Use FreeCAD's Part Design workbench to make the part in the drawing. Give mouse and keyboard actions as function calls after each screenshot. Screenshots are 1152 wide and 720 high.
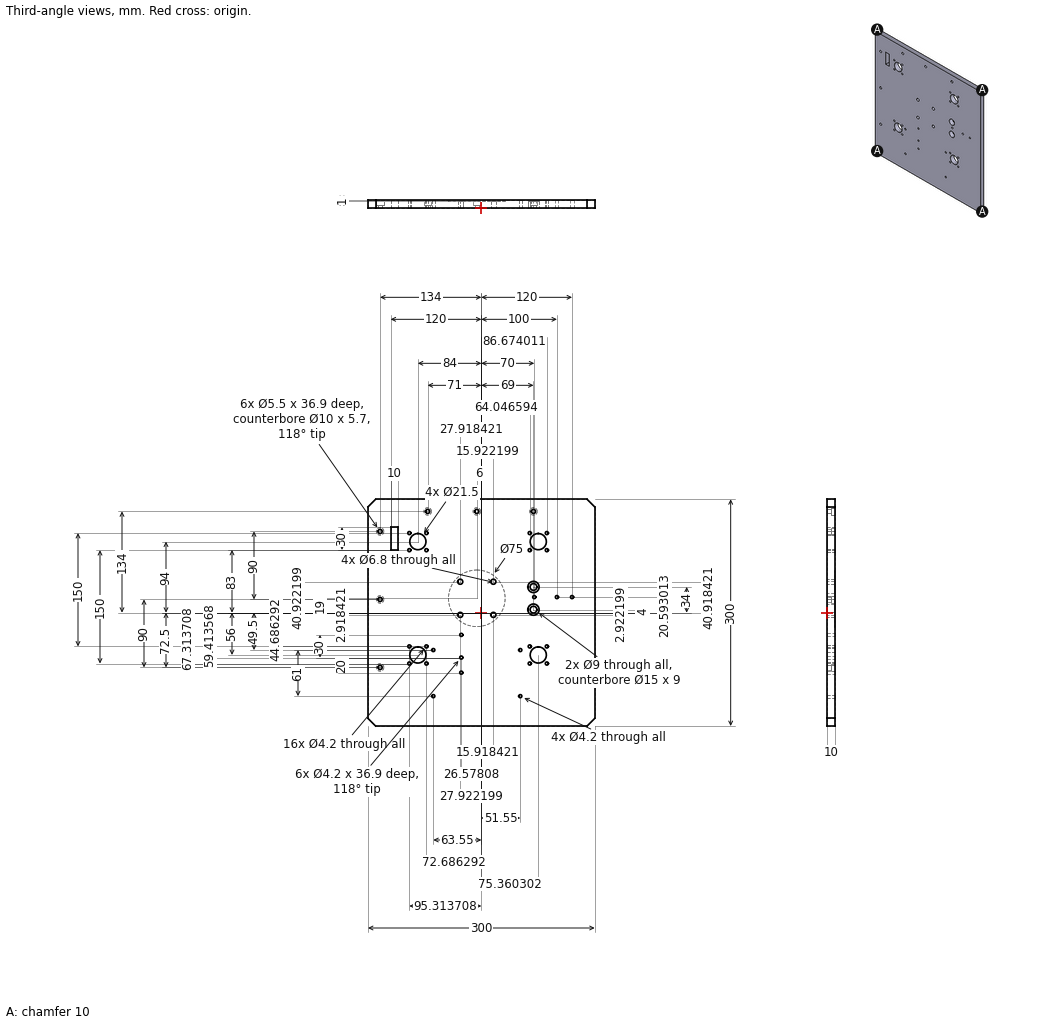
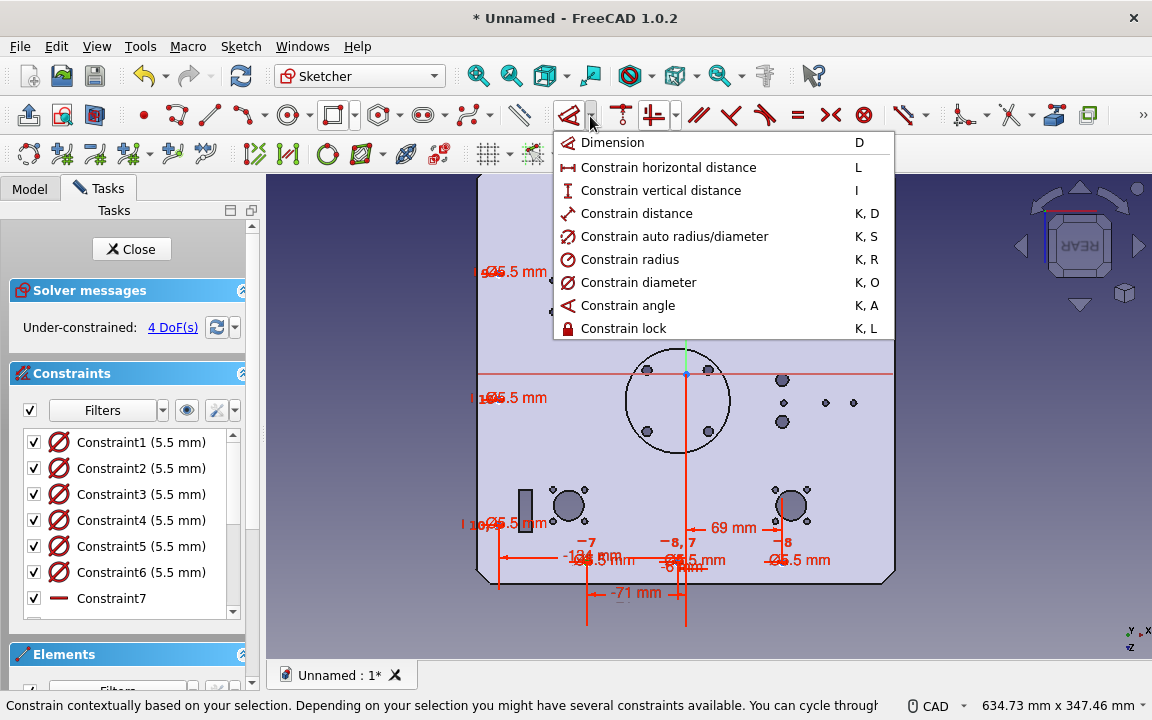
click(724, 190)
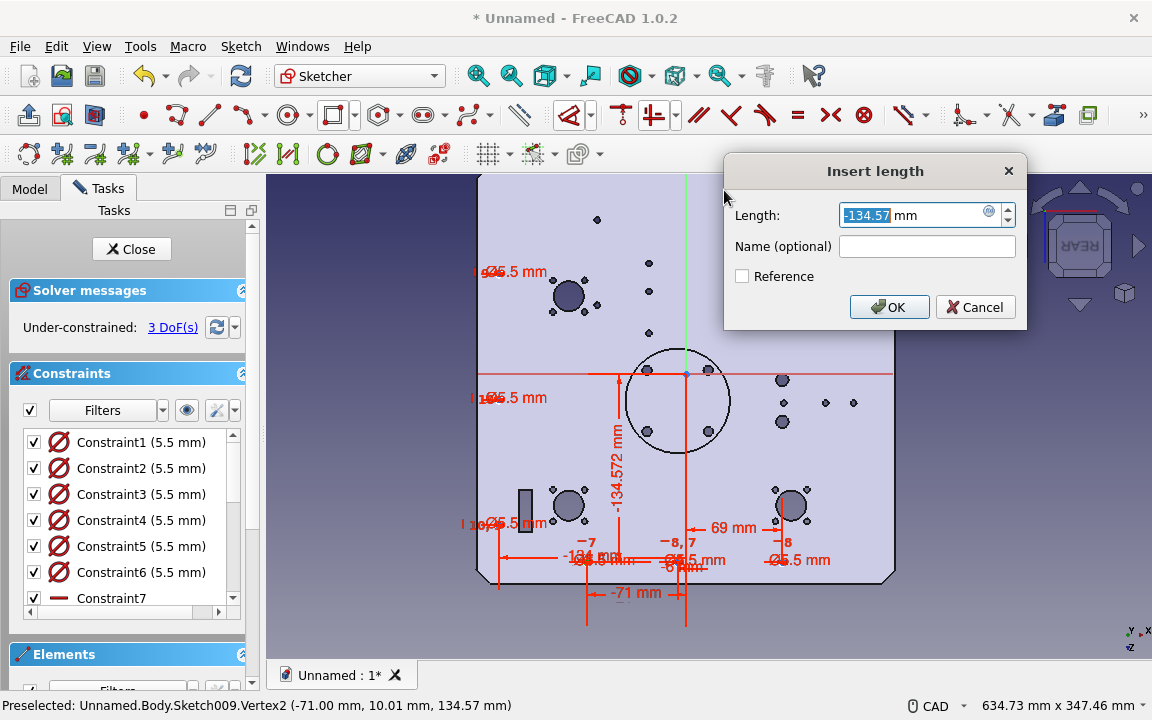
text(-134)
key(Return)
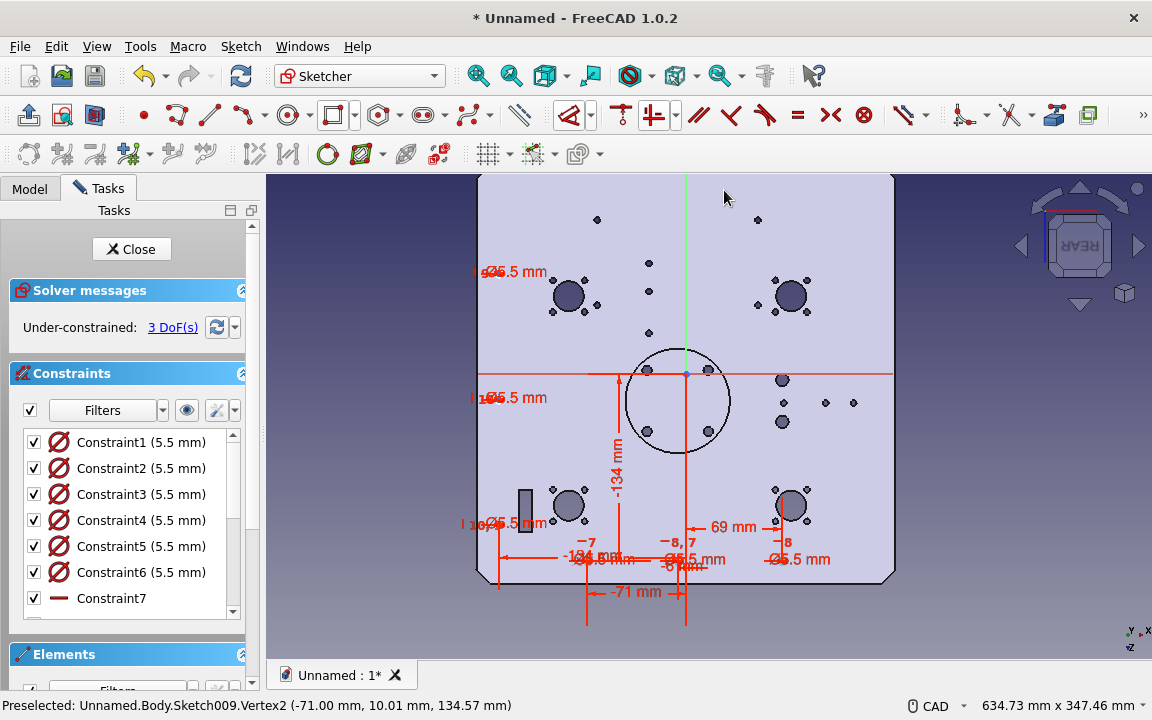
click(499, 525)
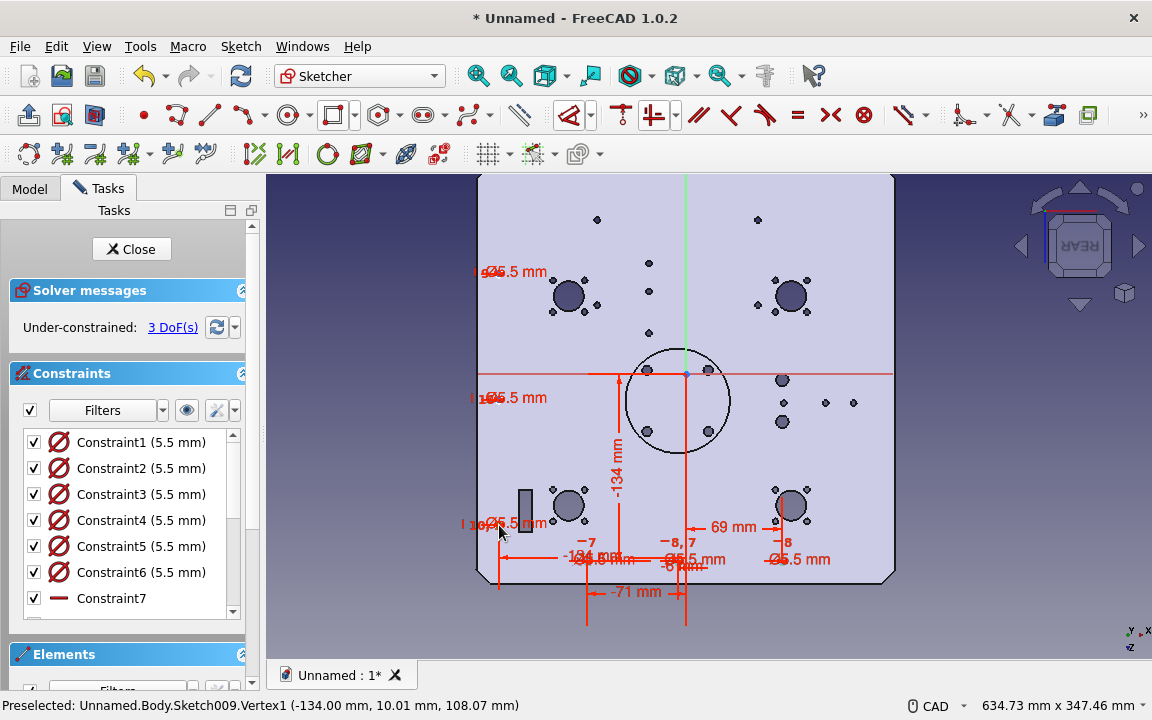
click(499, 400)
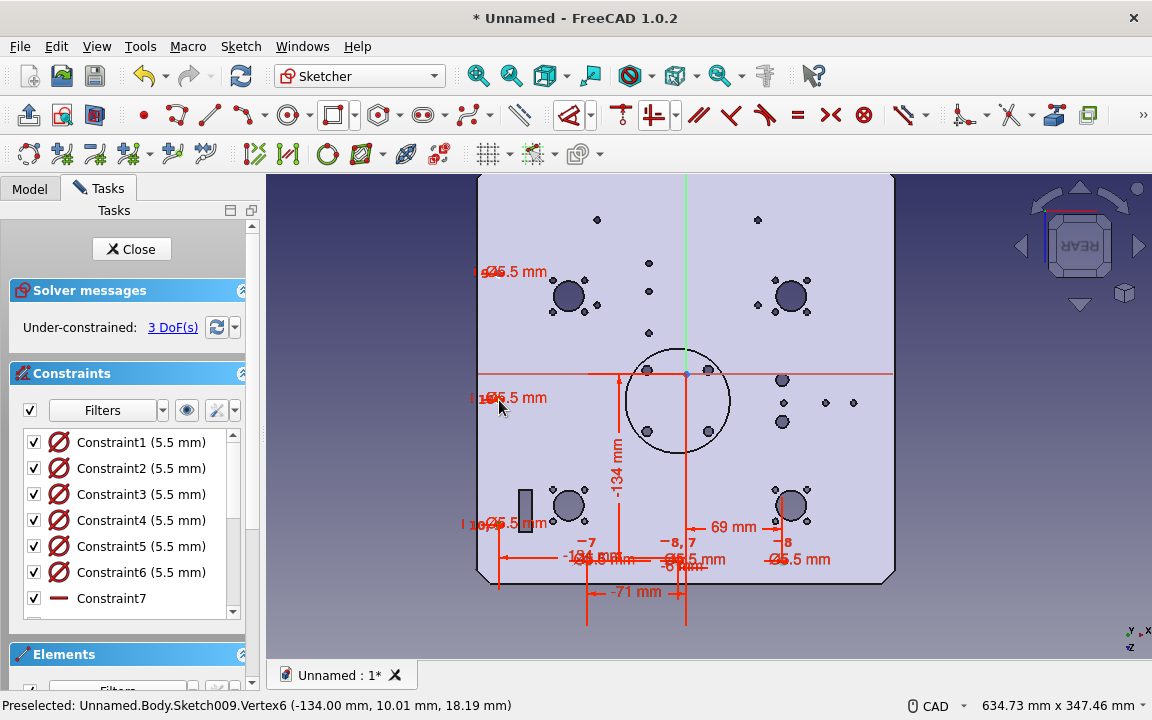
click(590, 116)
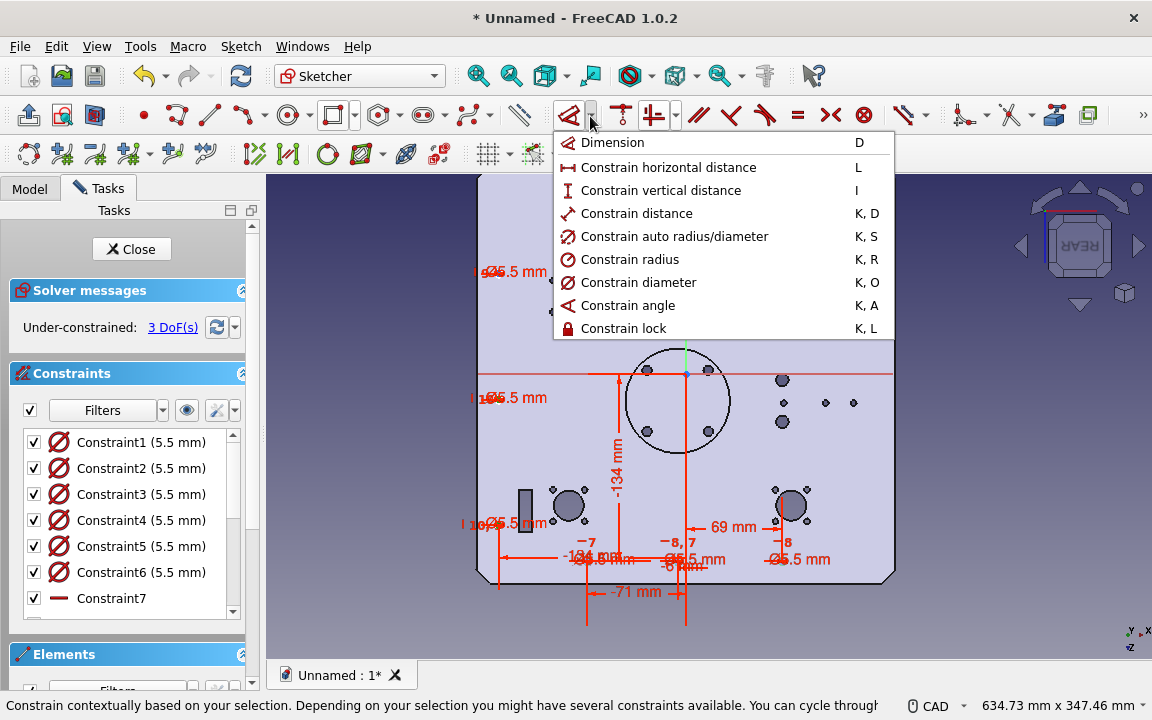
click(724, 190)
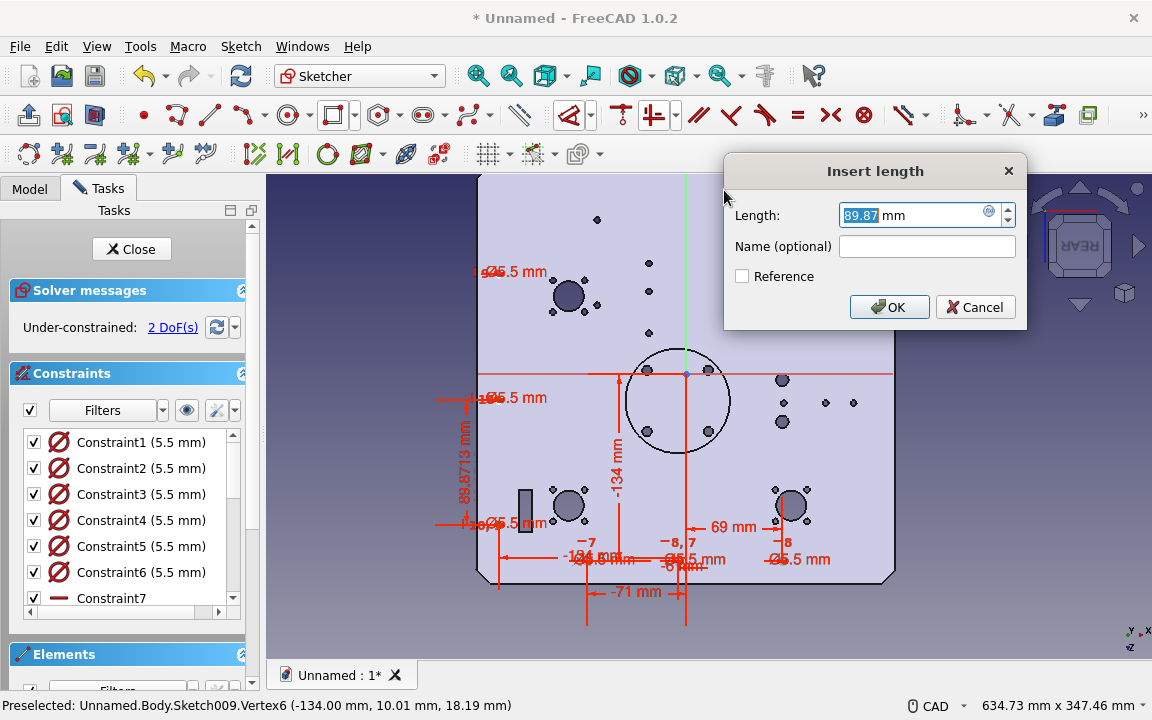
text(90)
key(Return)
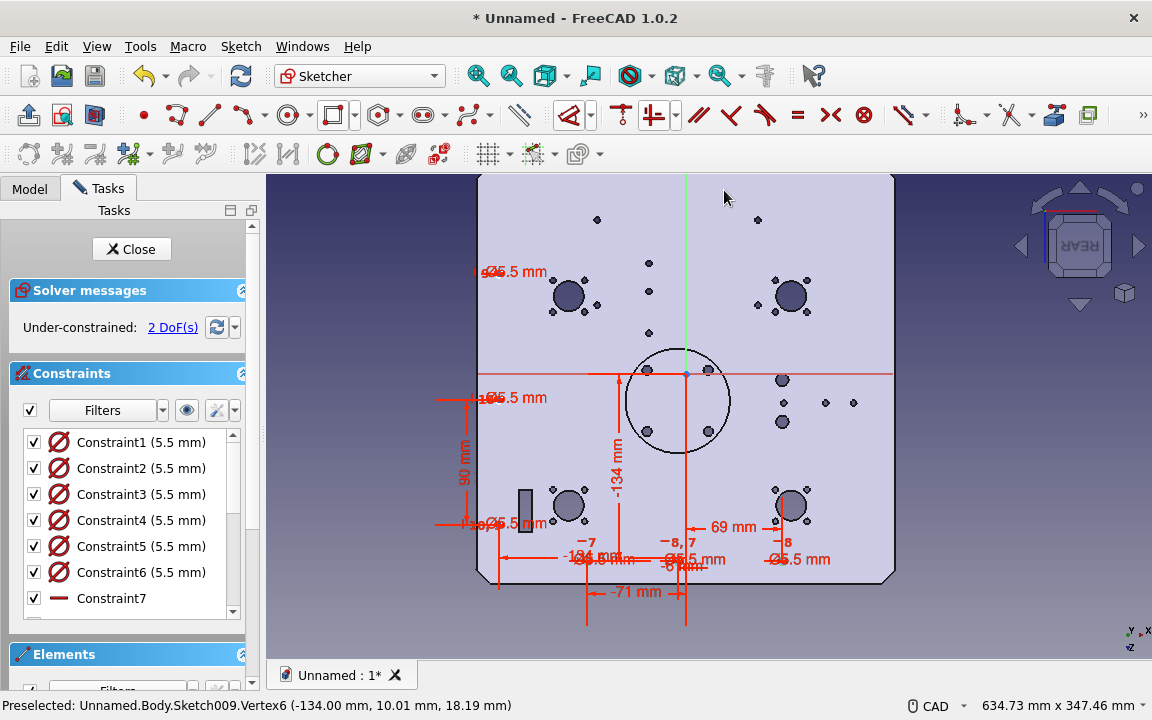
click(499, 274)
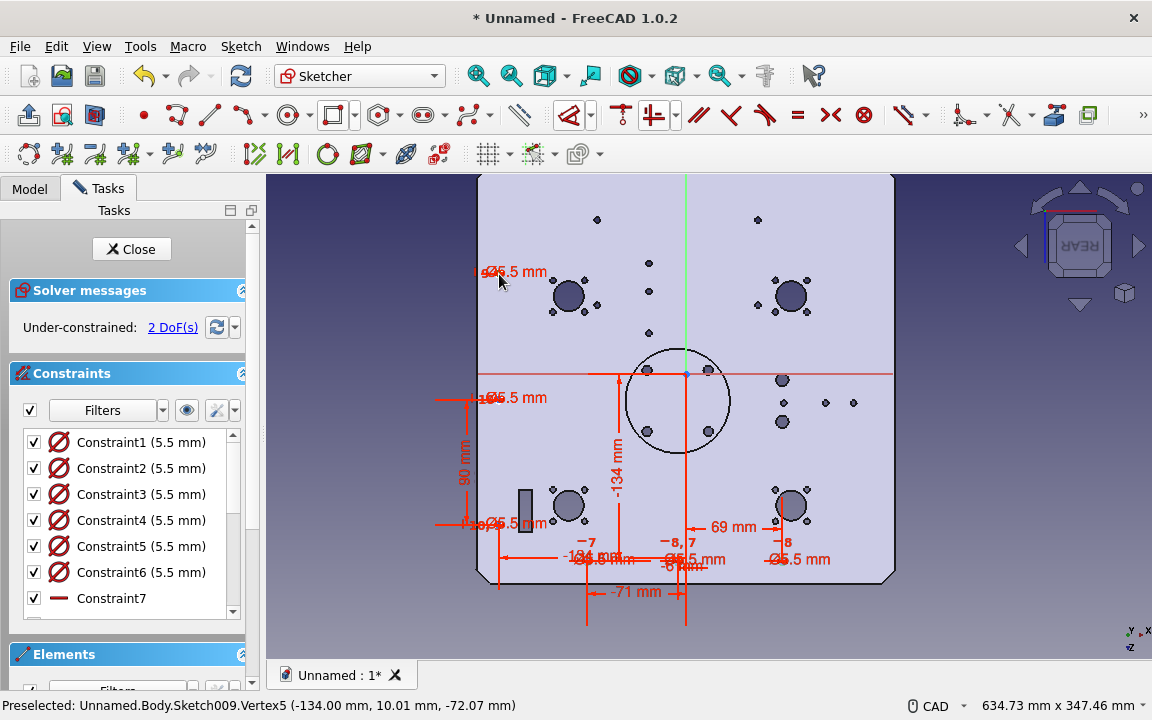
click(499, 400)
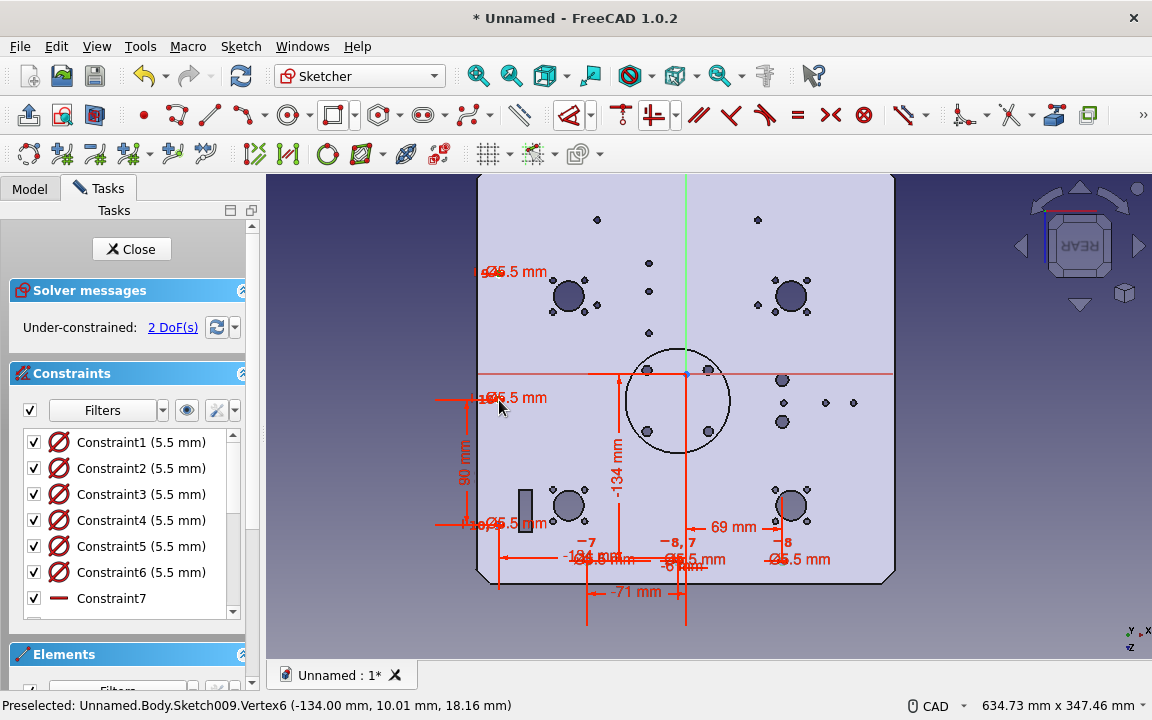
key(i)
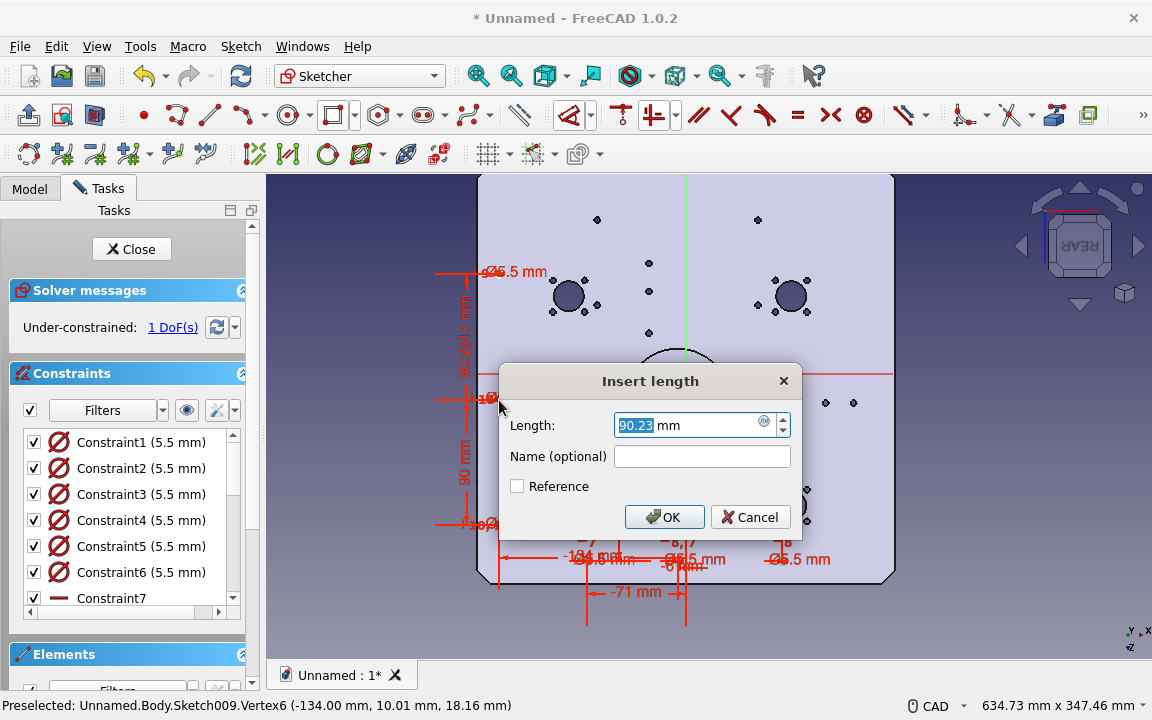
text(90)
key(Return)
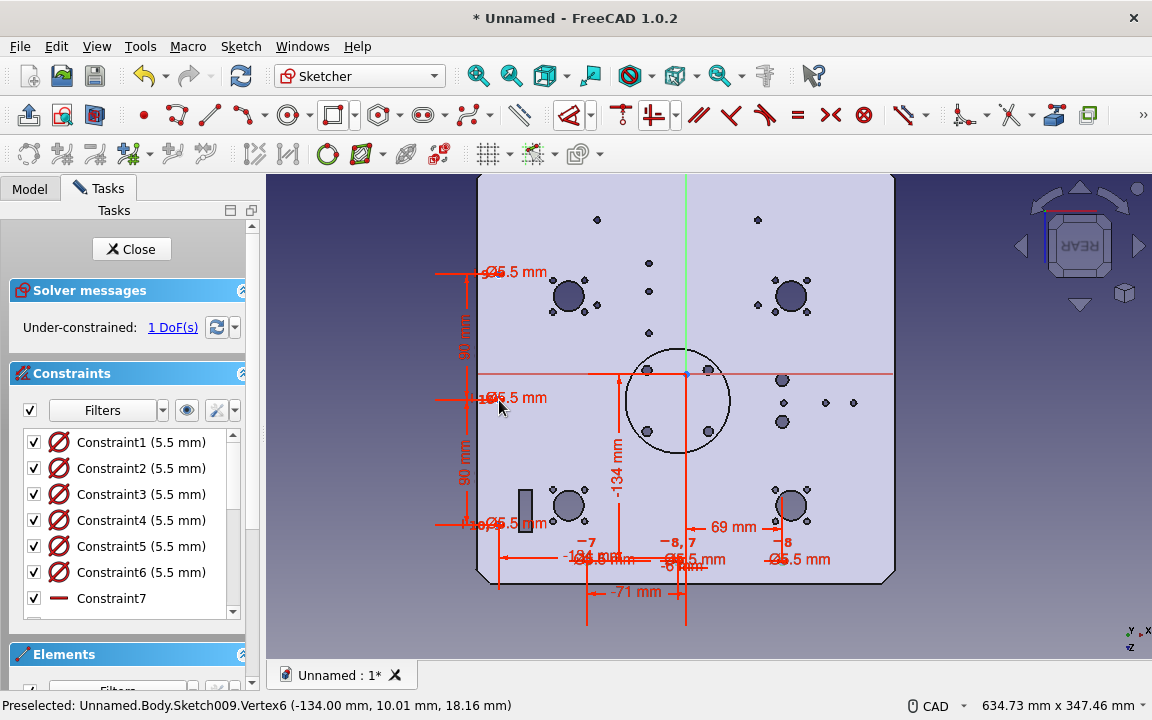
click(499, 274)